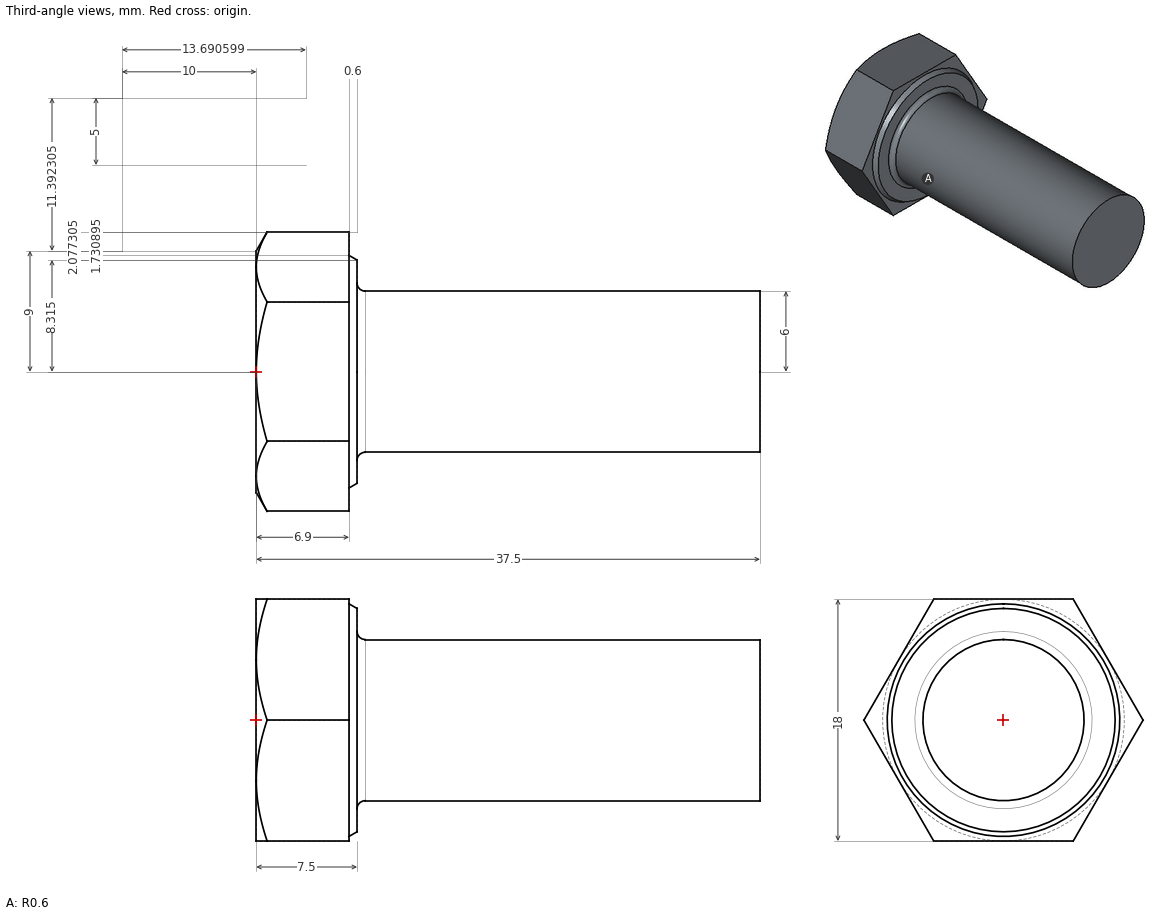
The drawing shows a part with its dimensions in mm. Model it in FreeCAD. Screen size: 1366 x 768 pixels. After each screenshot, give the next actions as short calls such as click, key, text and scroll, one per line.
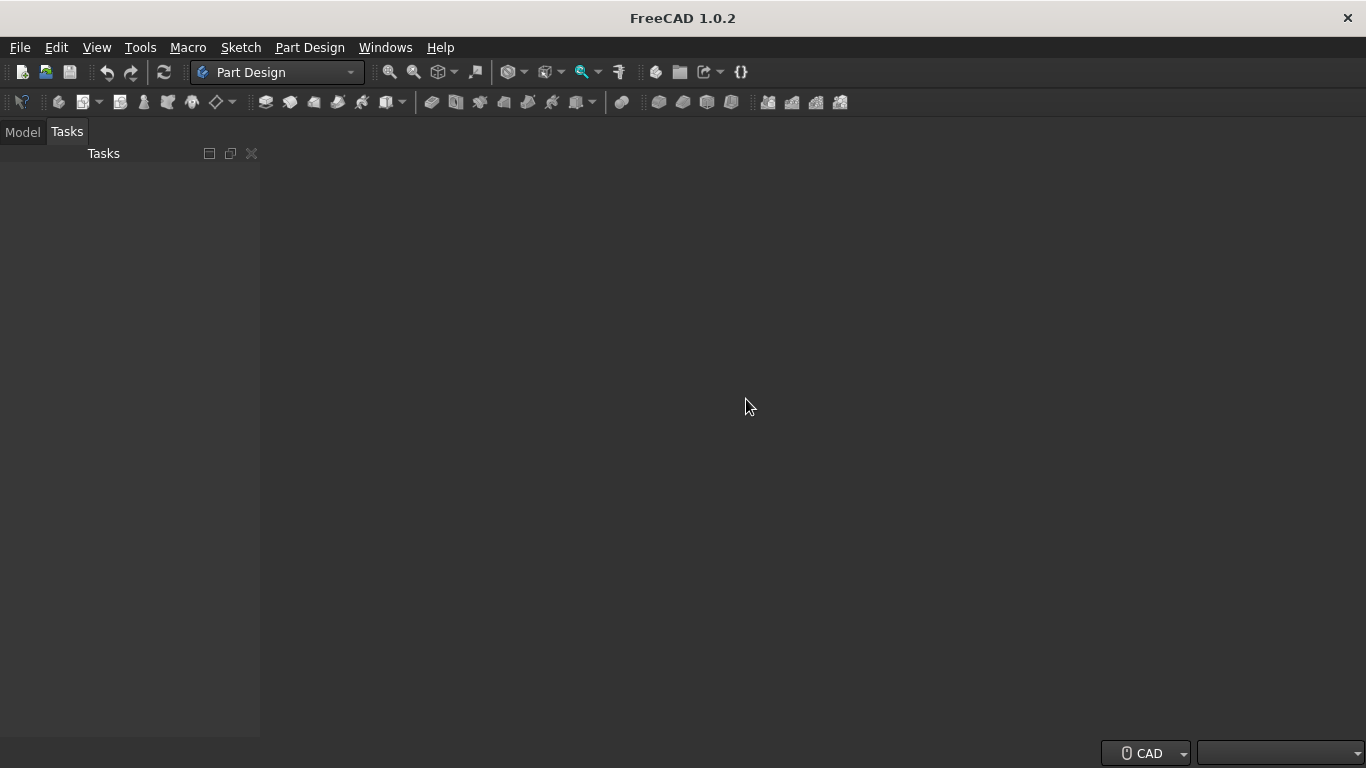
key(ctrl+n)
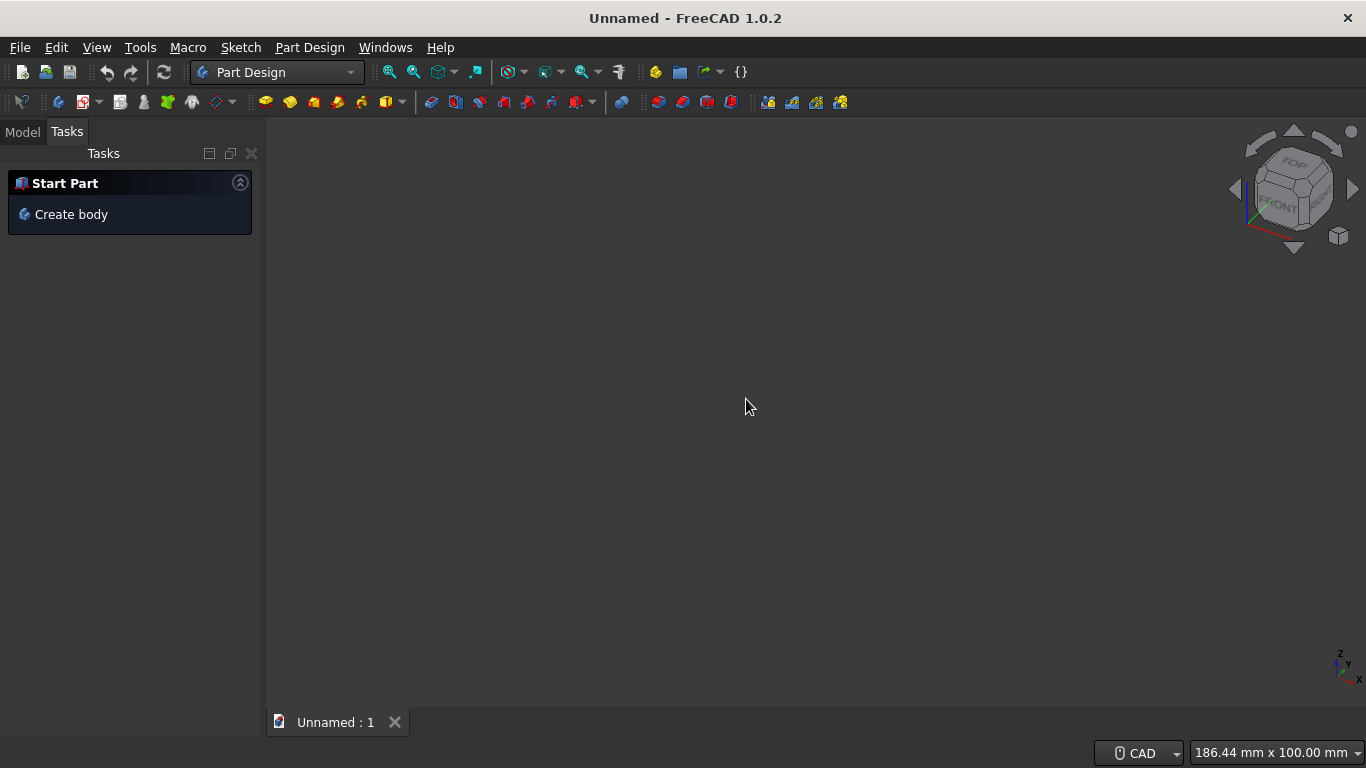
click(84, 102)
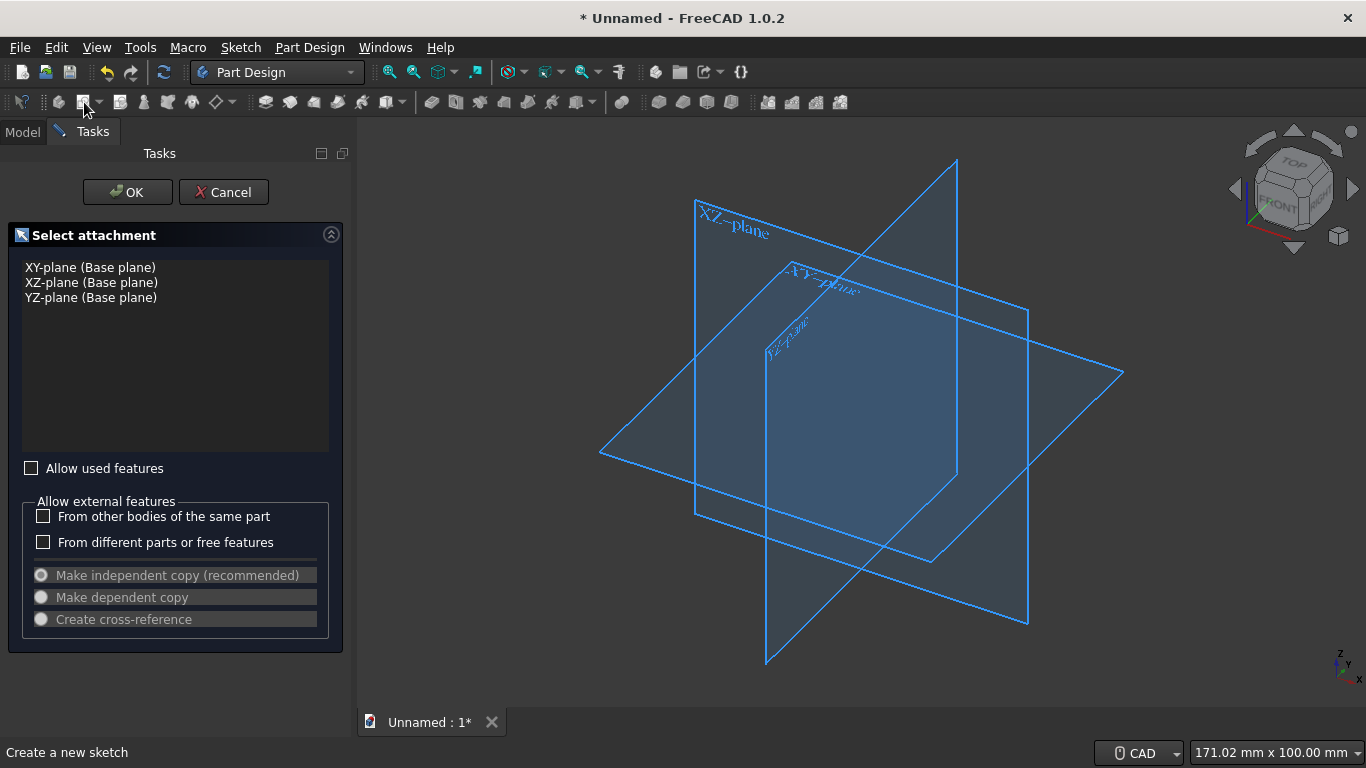
click(82, 298)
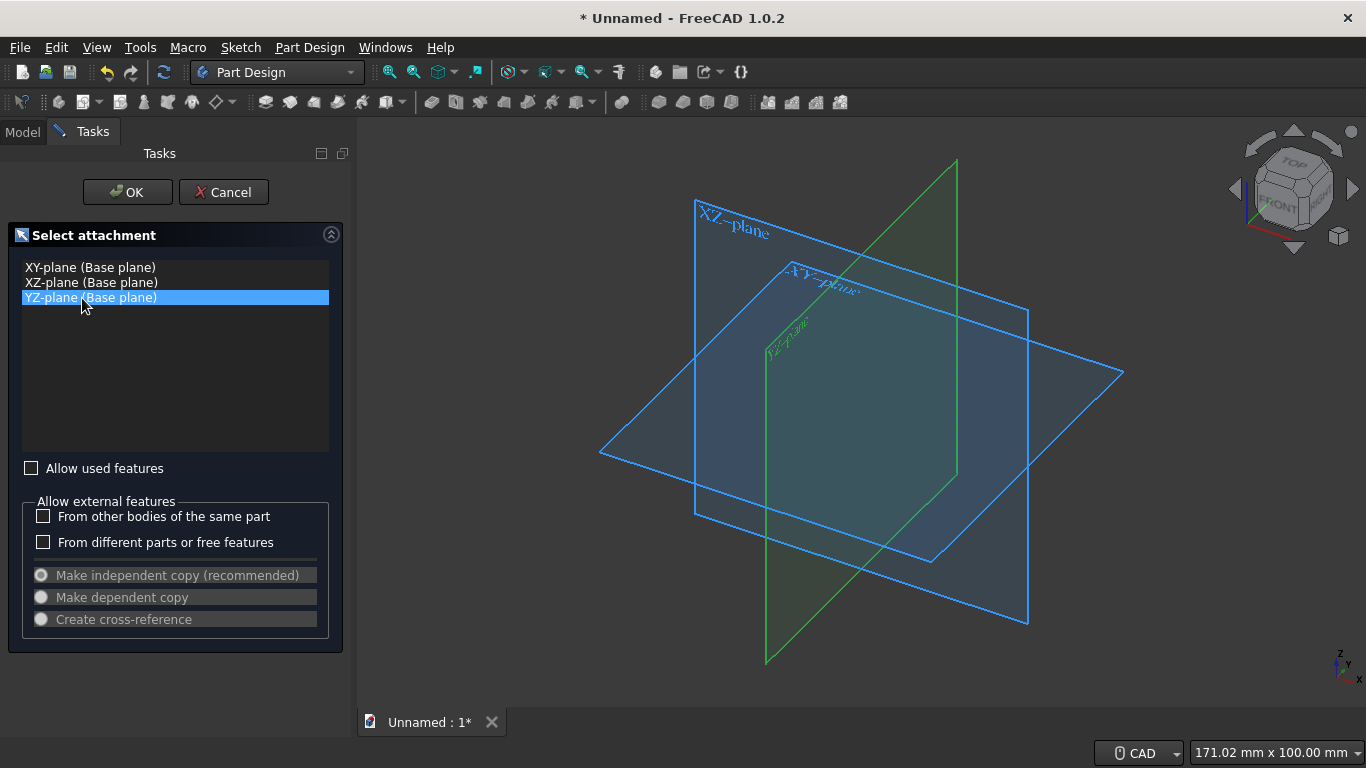
click(128, 192)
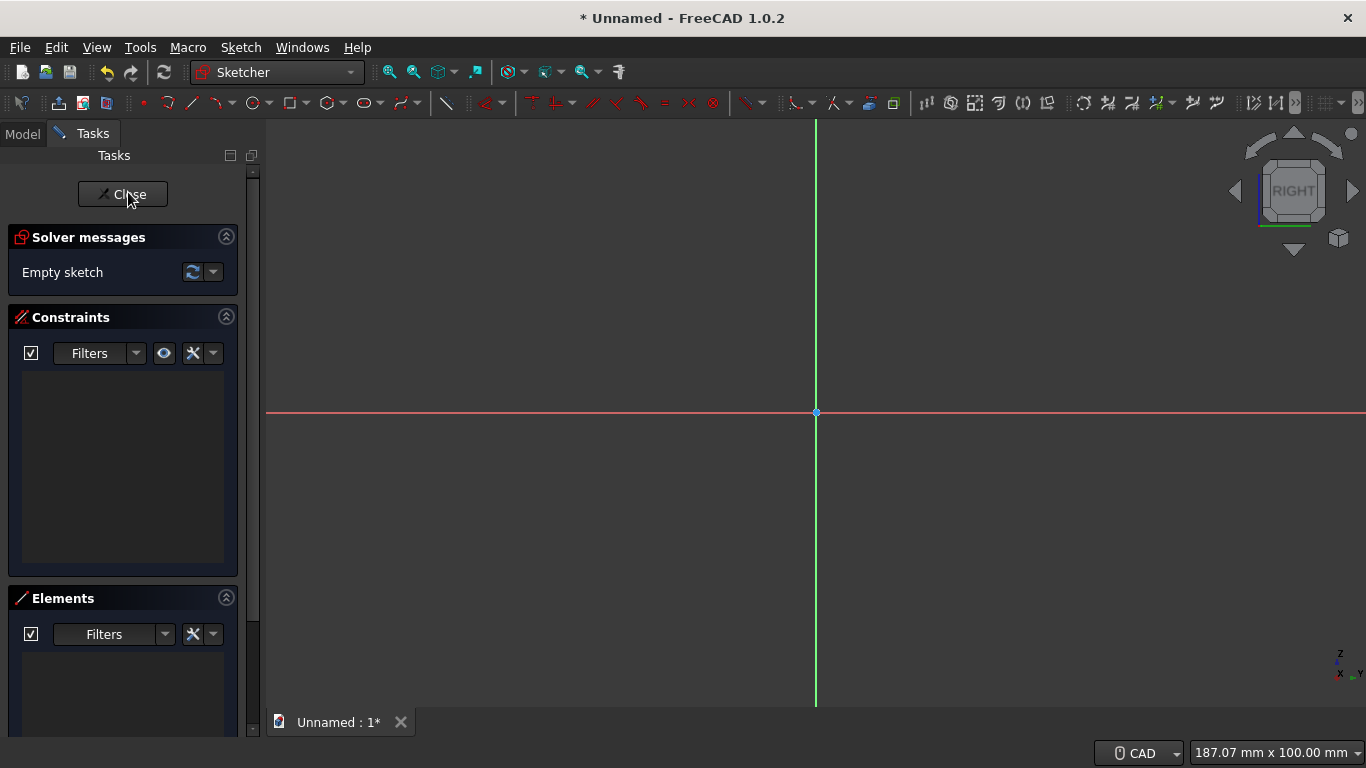
scroll(846, 413, up, 6)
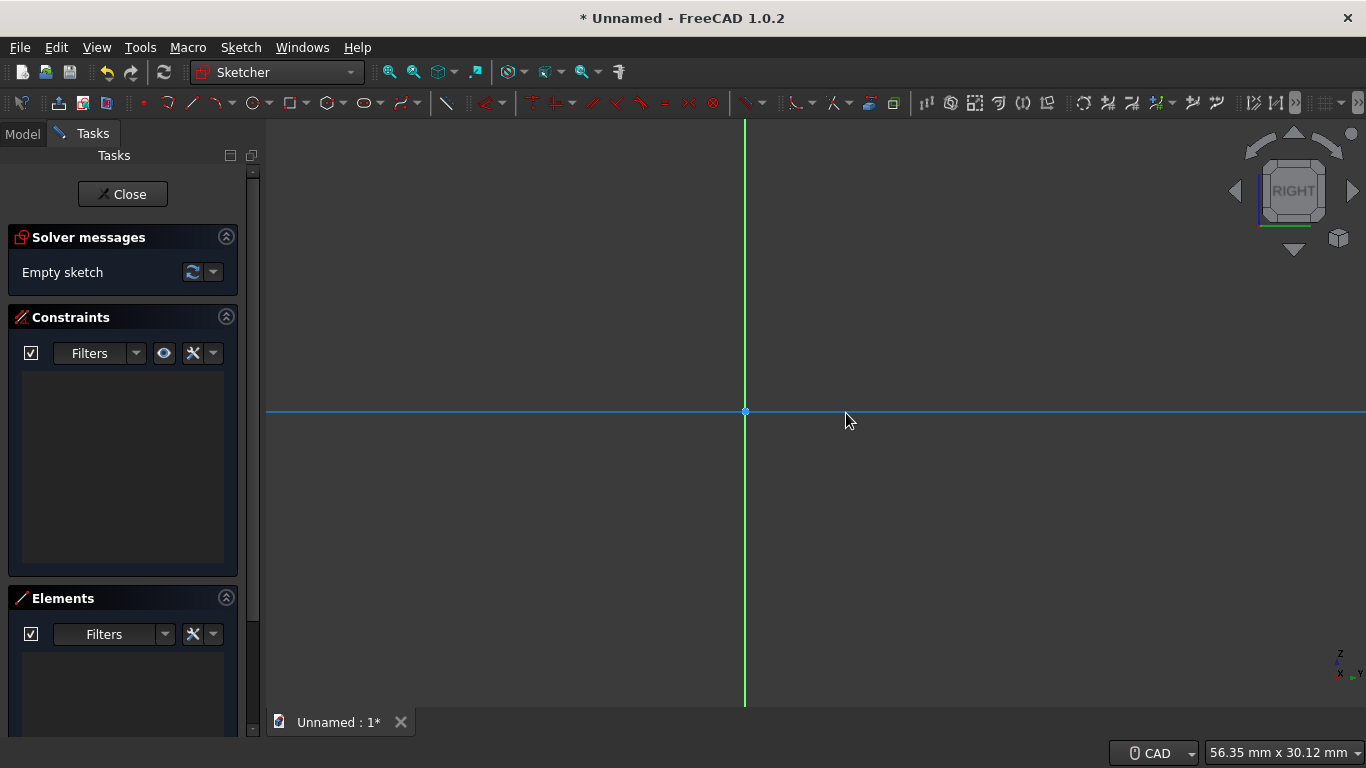
click(328, 104)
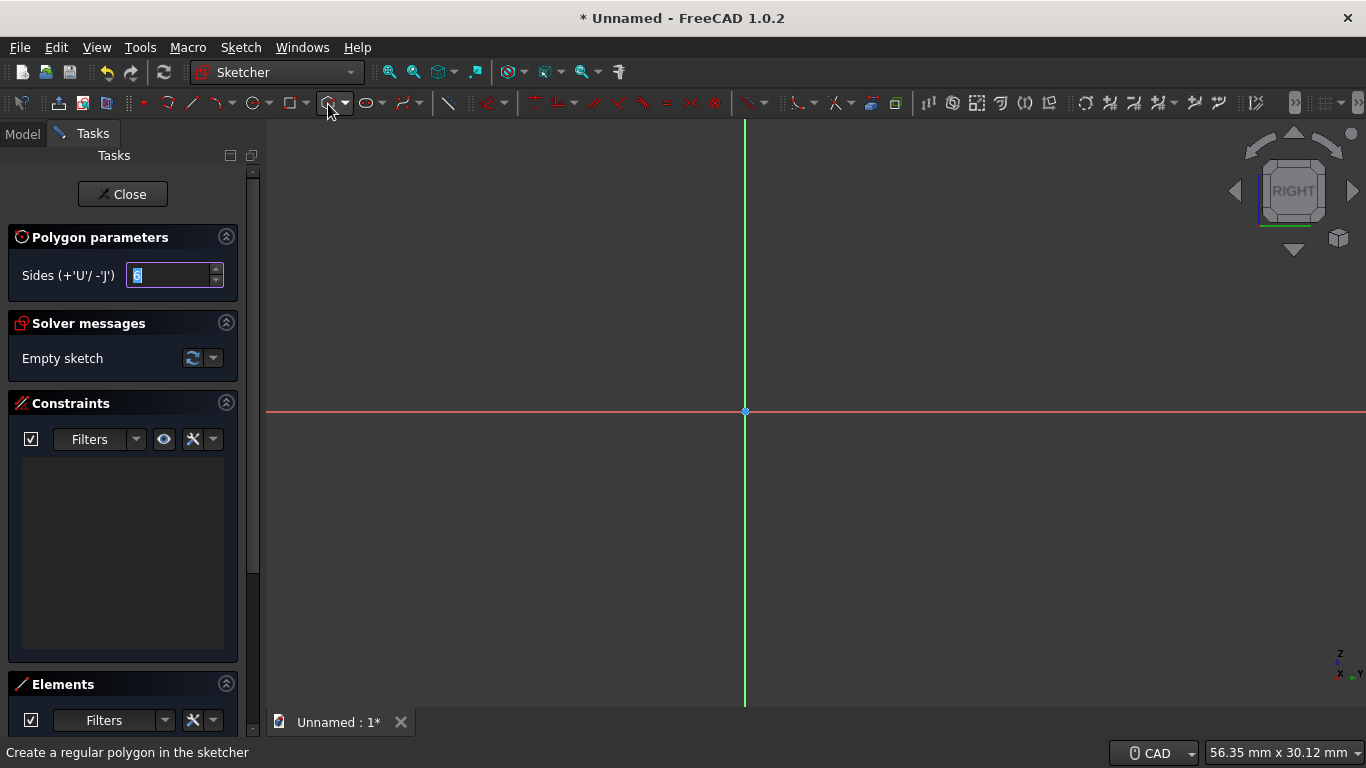
click(745, 412)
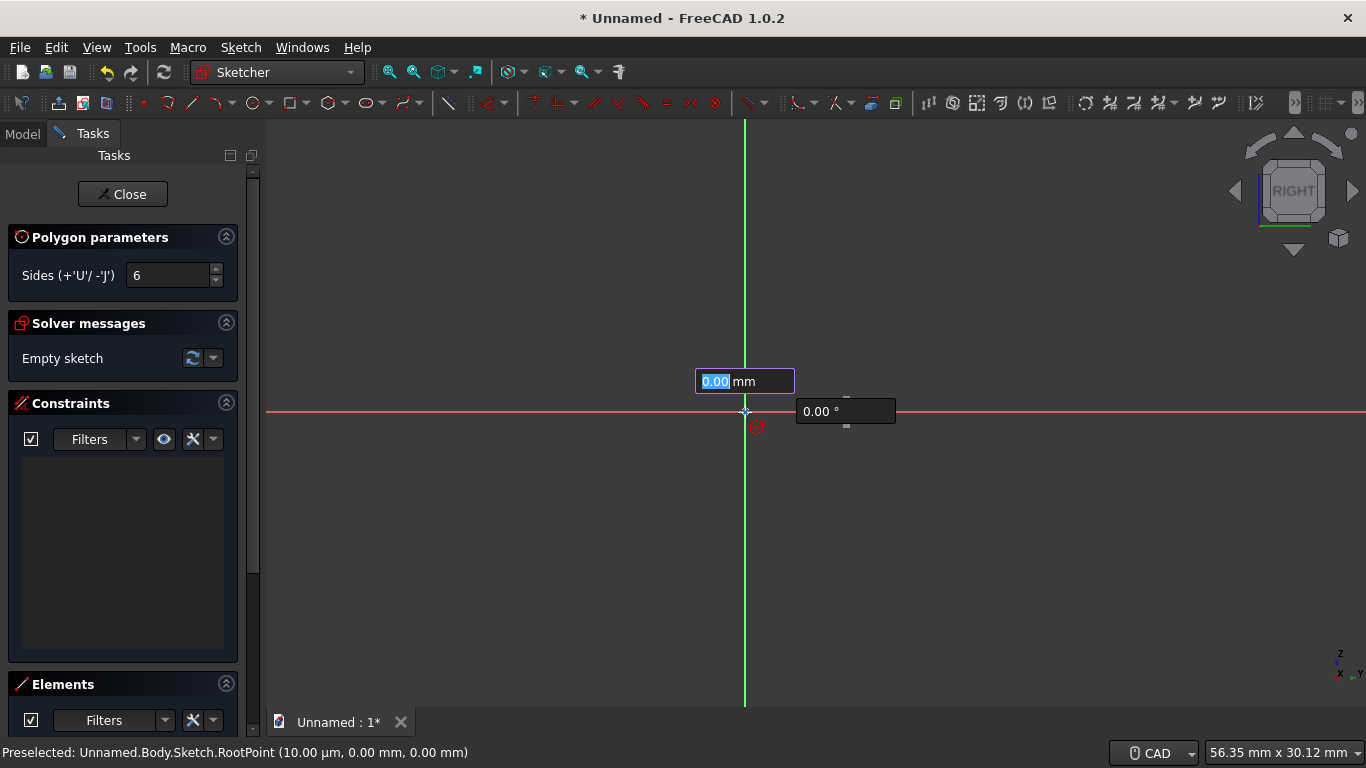
click(948, 412)
right_click(948, 412)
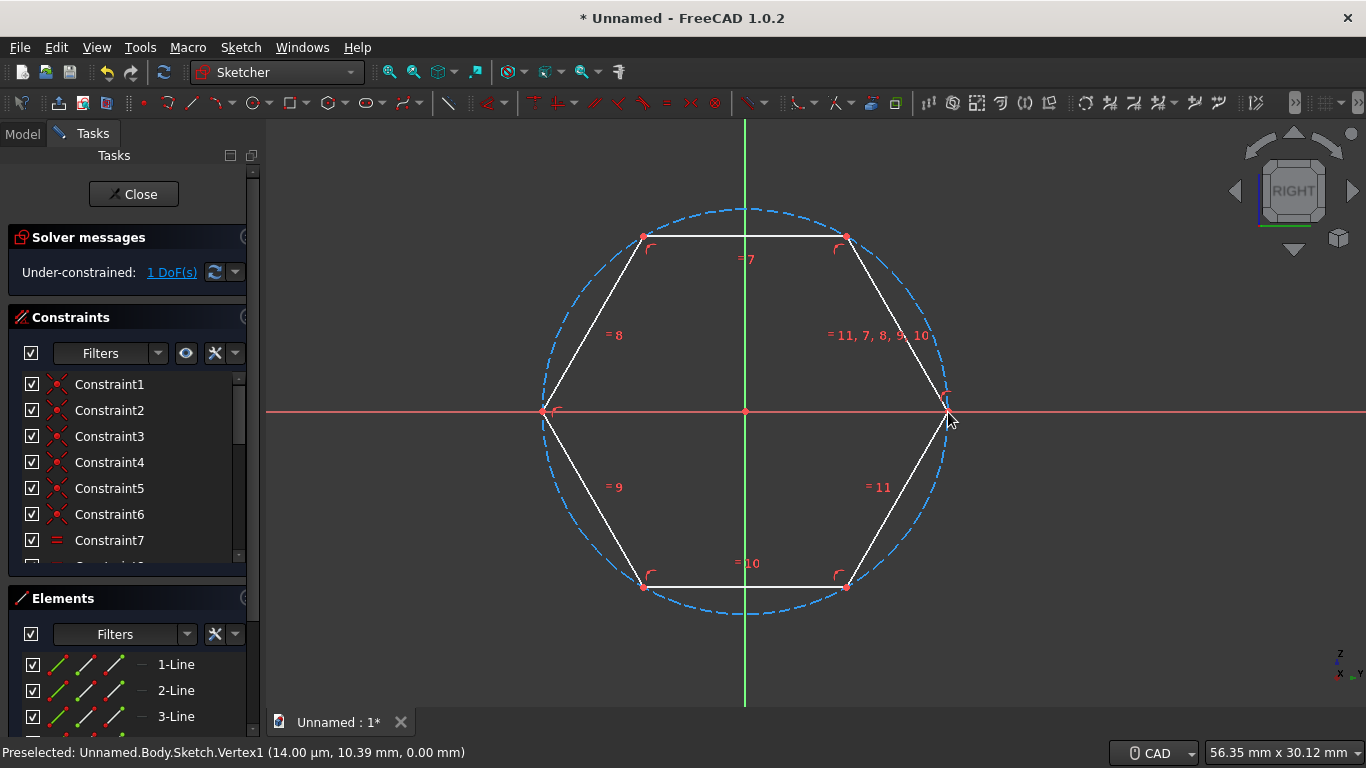
click(644, 587)